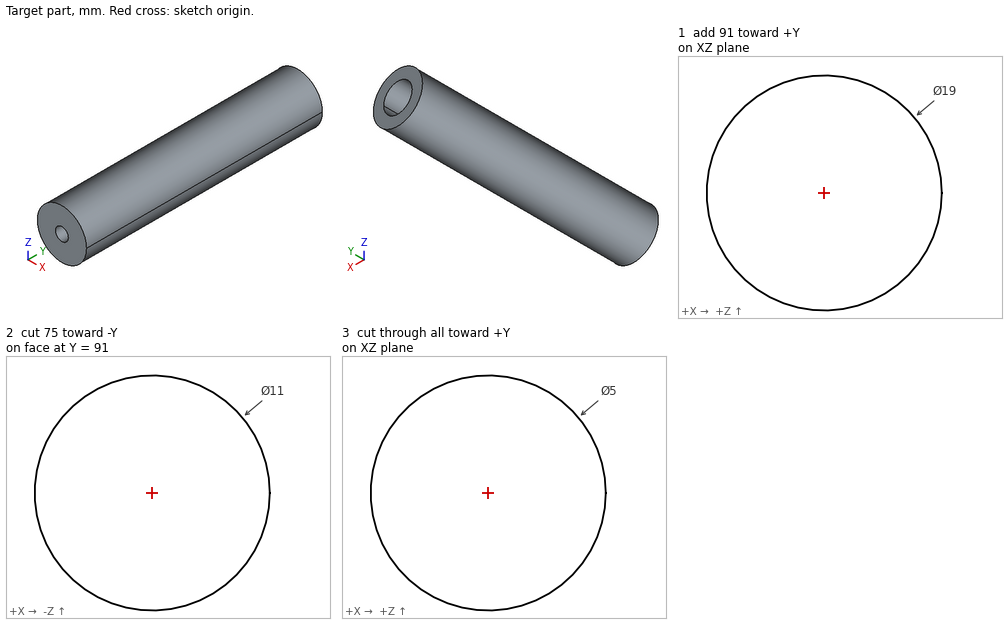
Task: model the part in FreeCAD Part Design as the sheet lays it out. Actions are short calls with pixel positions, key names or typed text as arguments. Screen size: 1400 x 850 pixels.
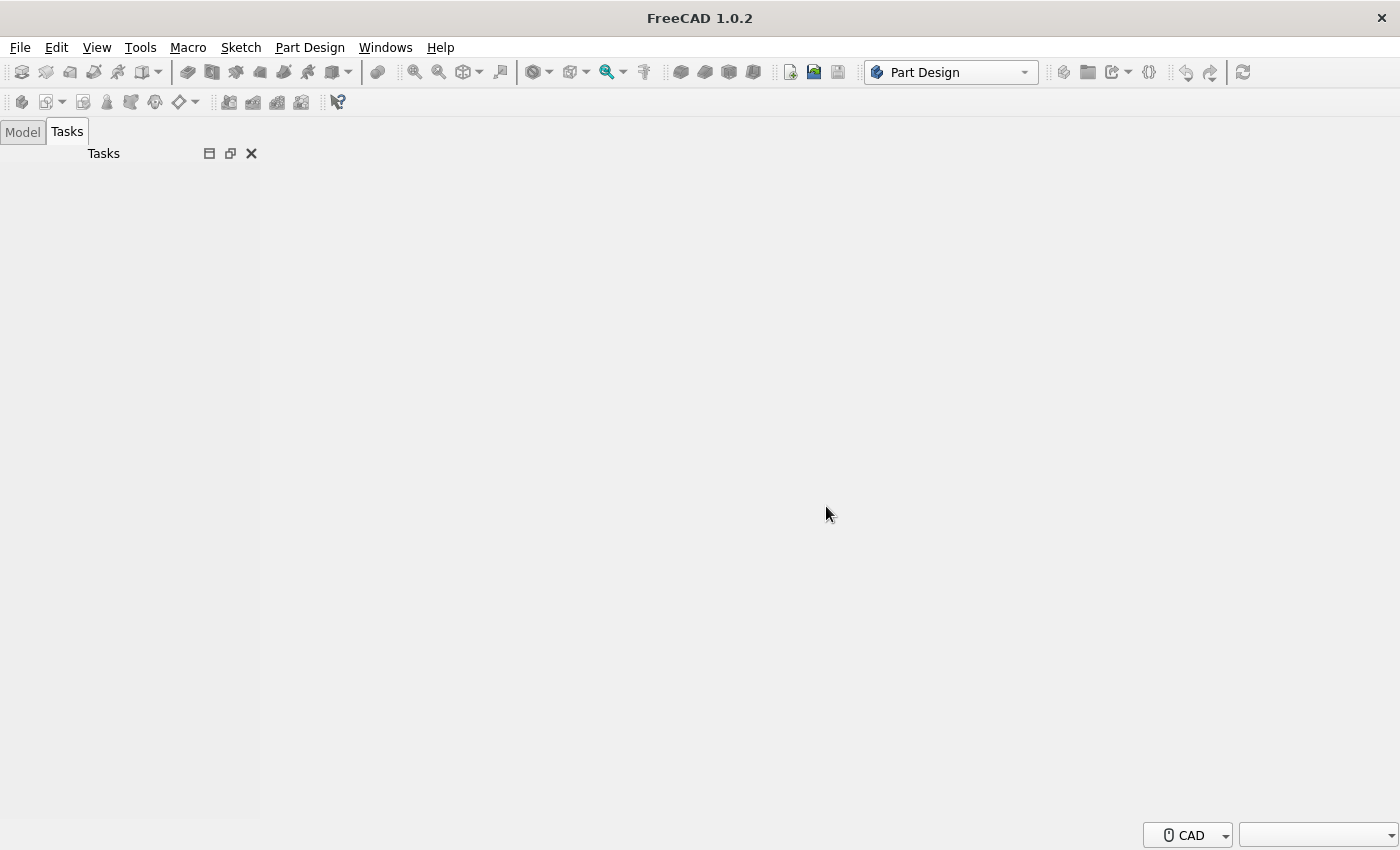
key(ctrl+n)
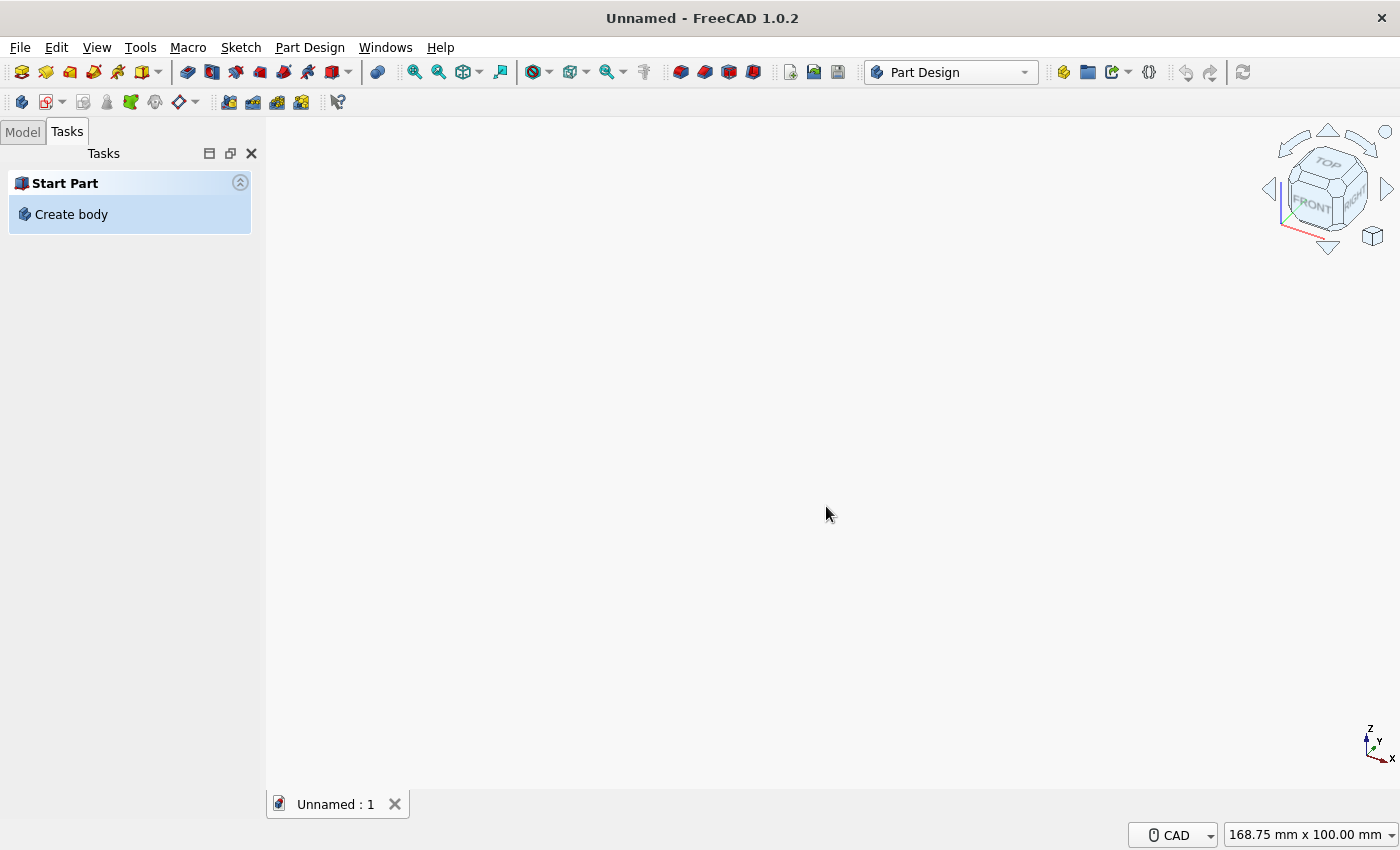
click(46, 102)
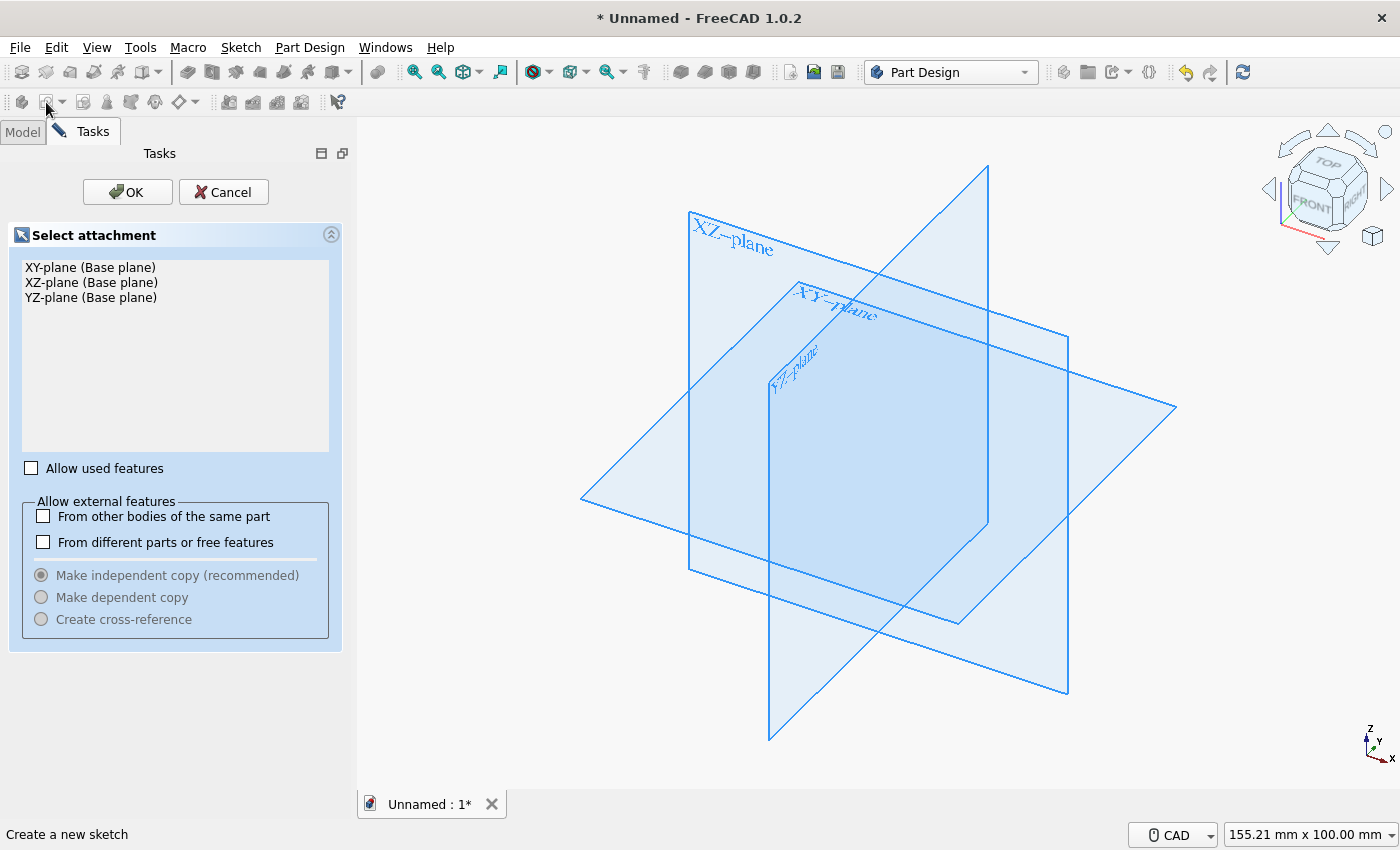
click(82, 282)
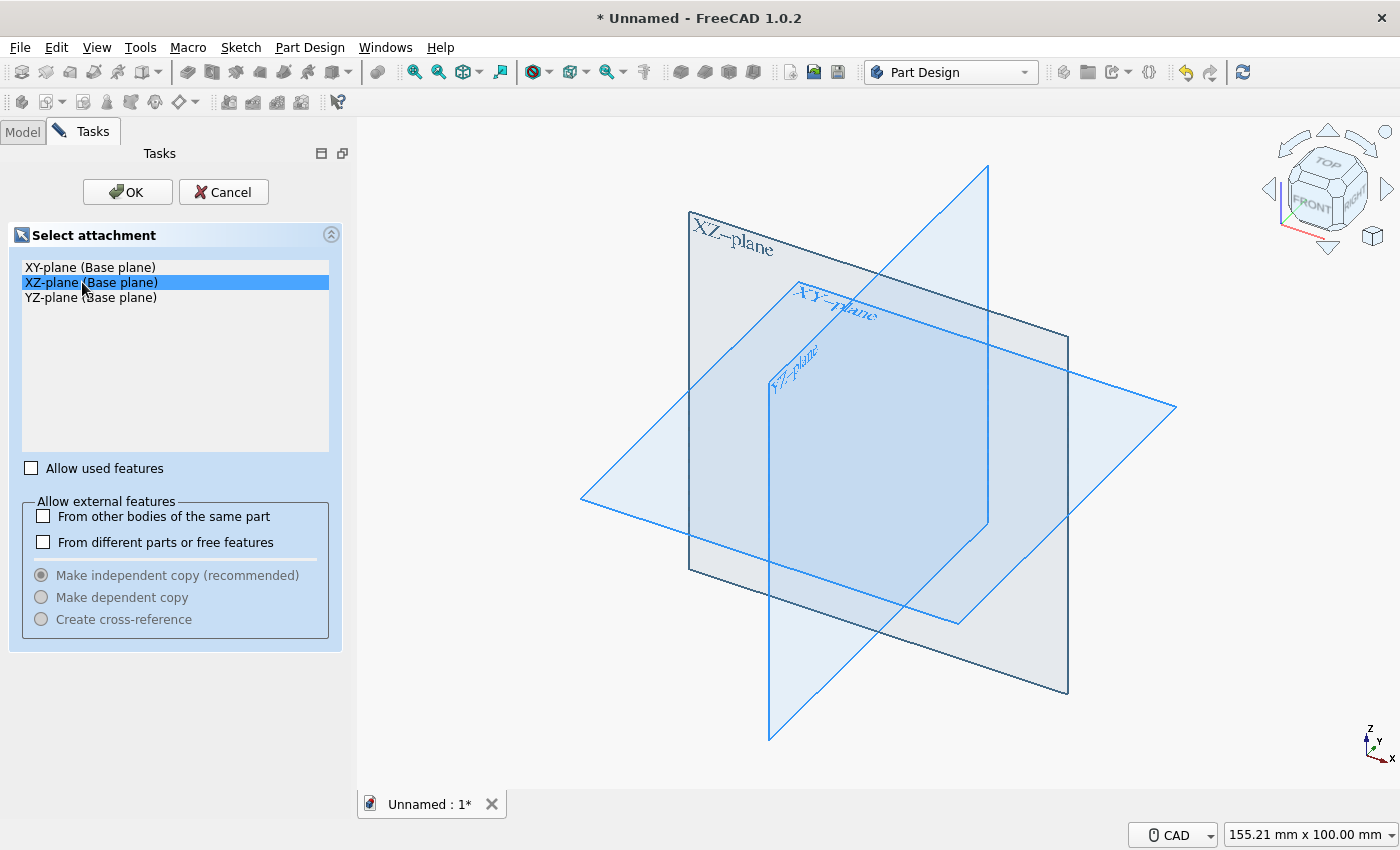
click(128, 192)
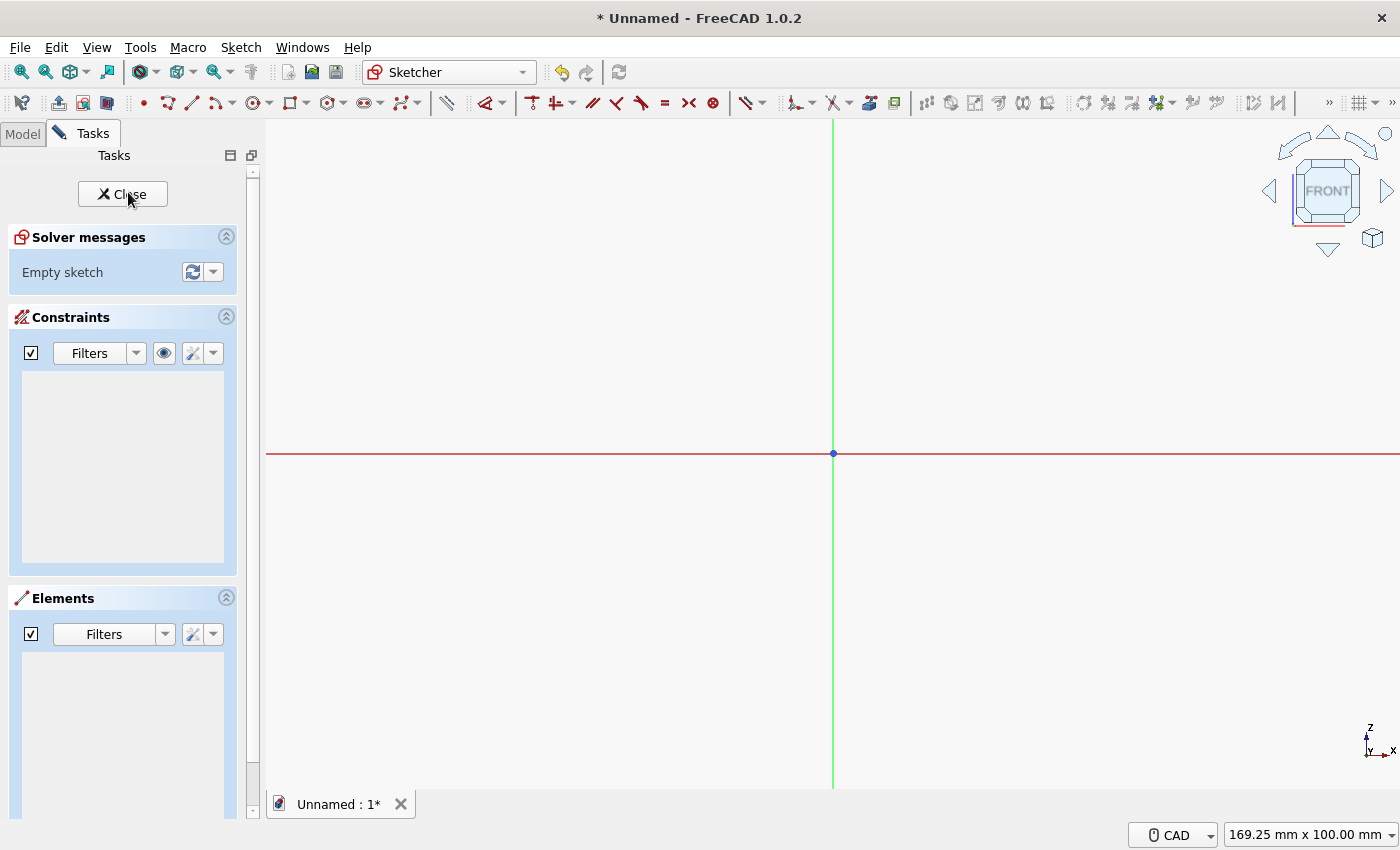
scroll(863, 454, up, 6)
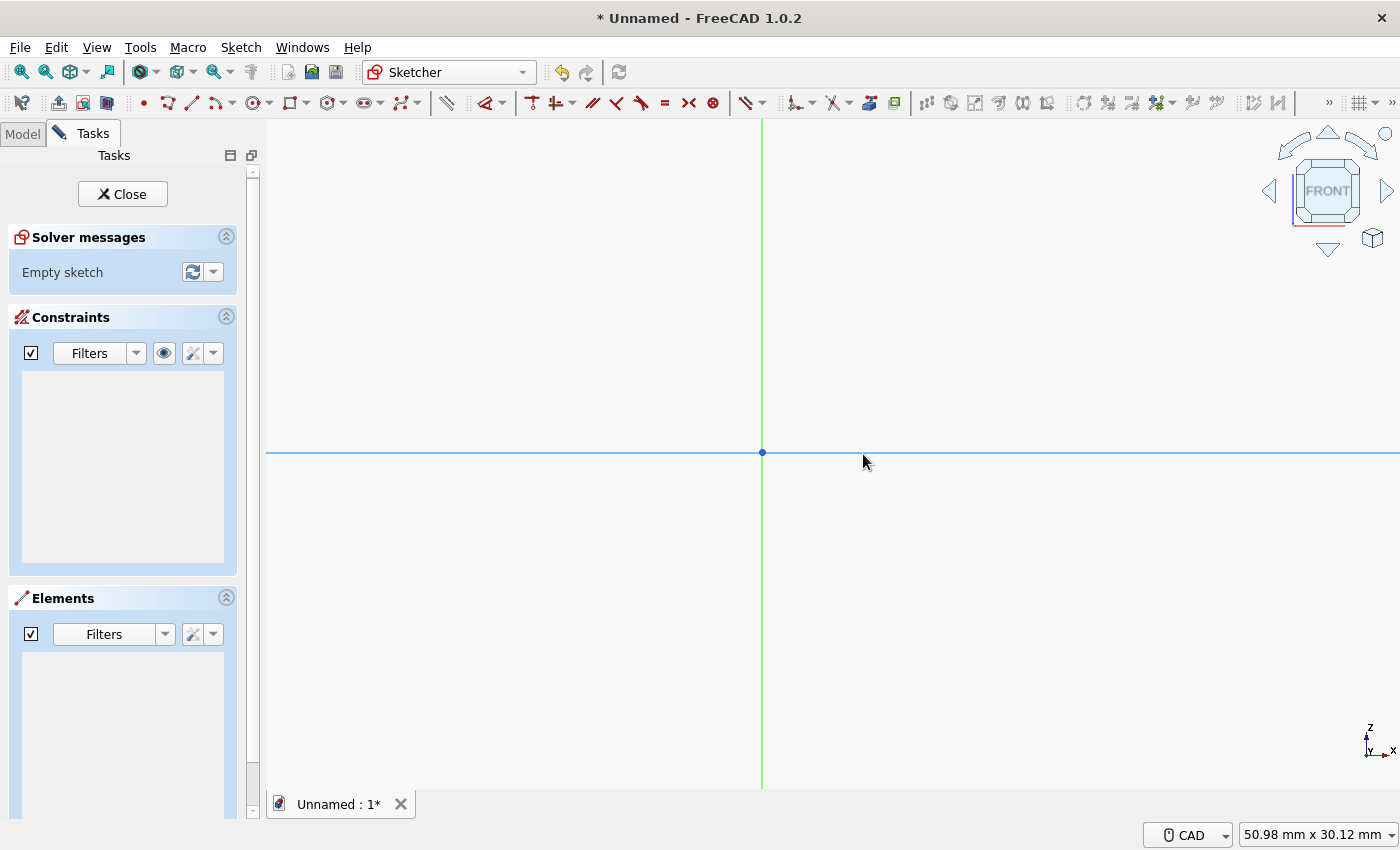
click(254, 104)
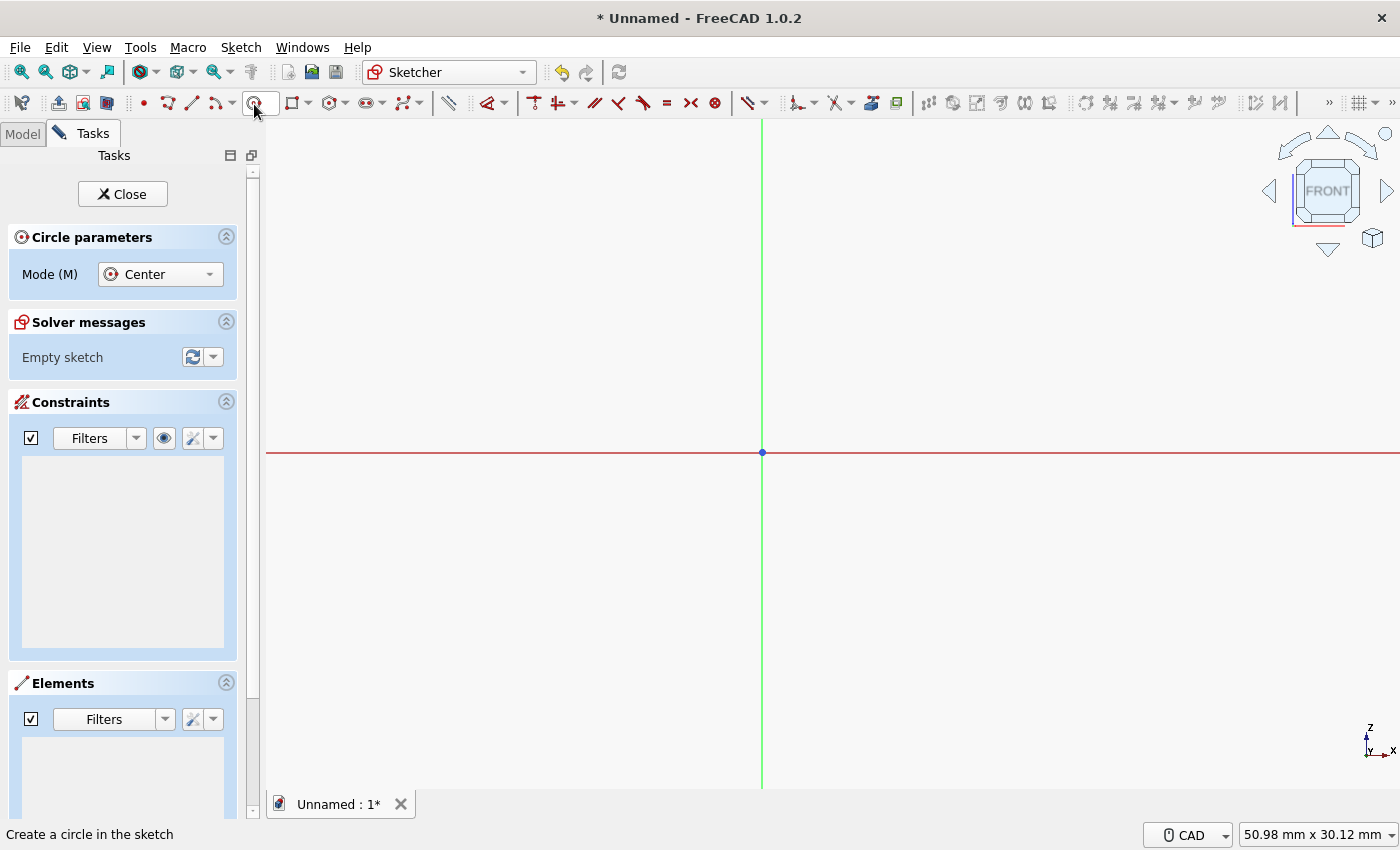
click(762, 453)
click(912, 303)
key(Escape)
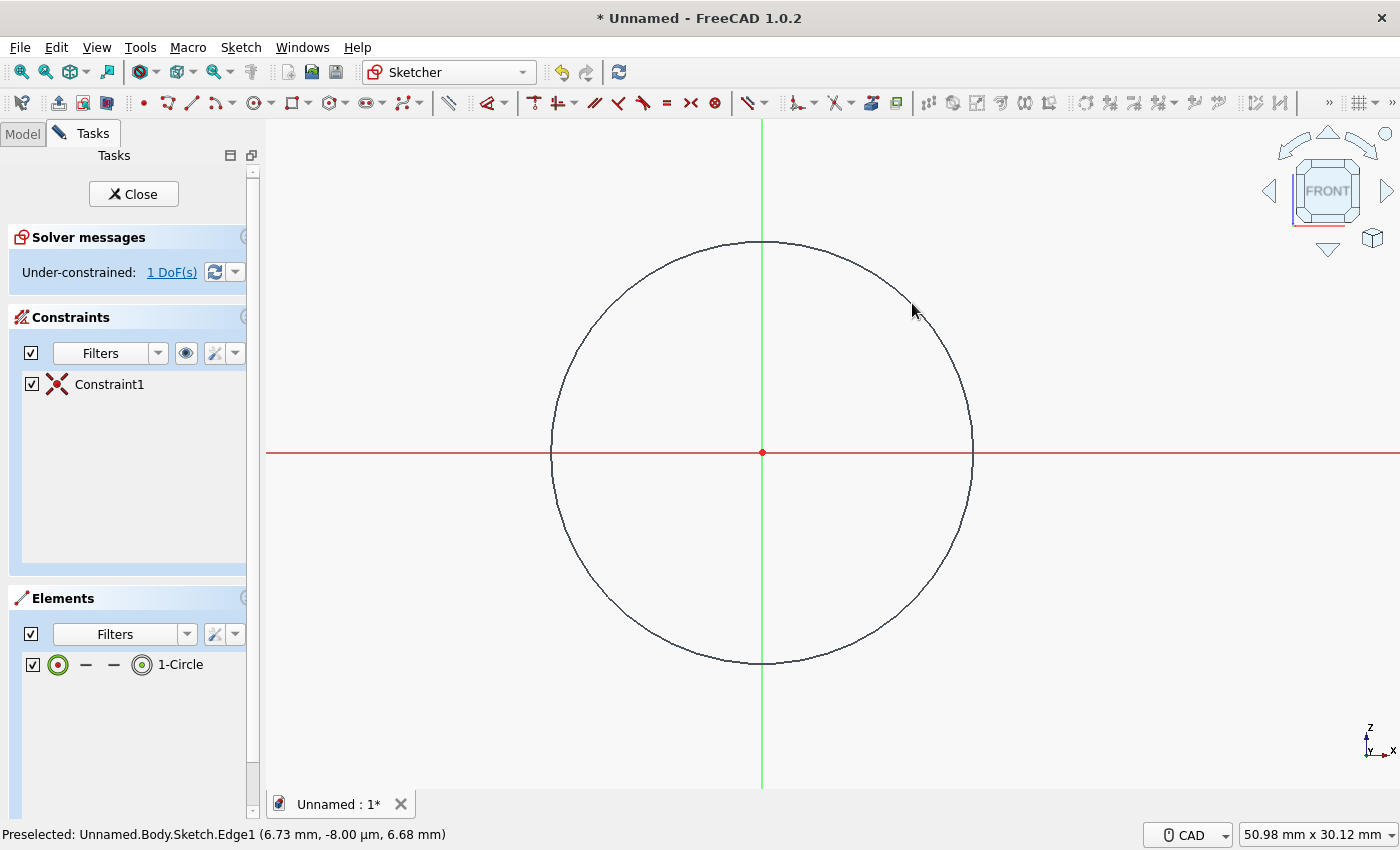
click(911, 303)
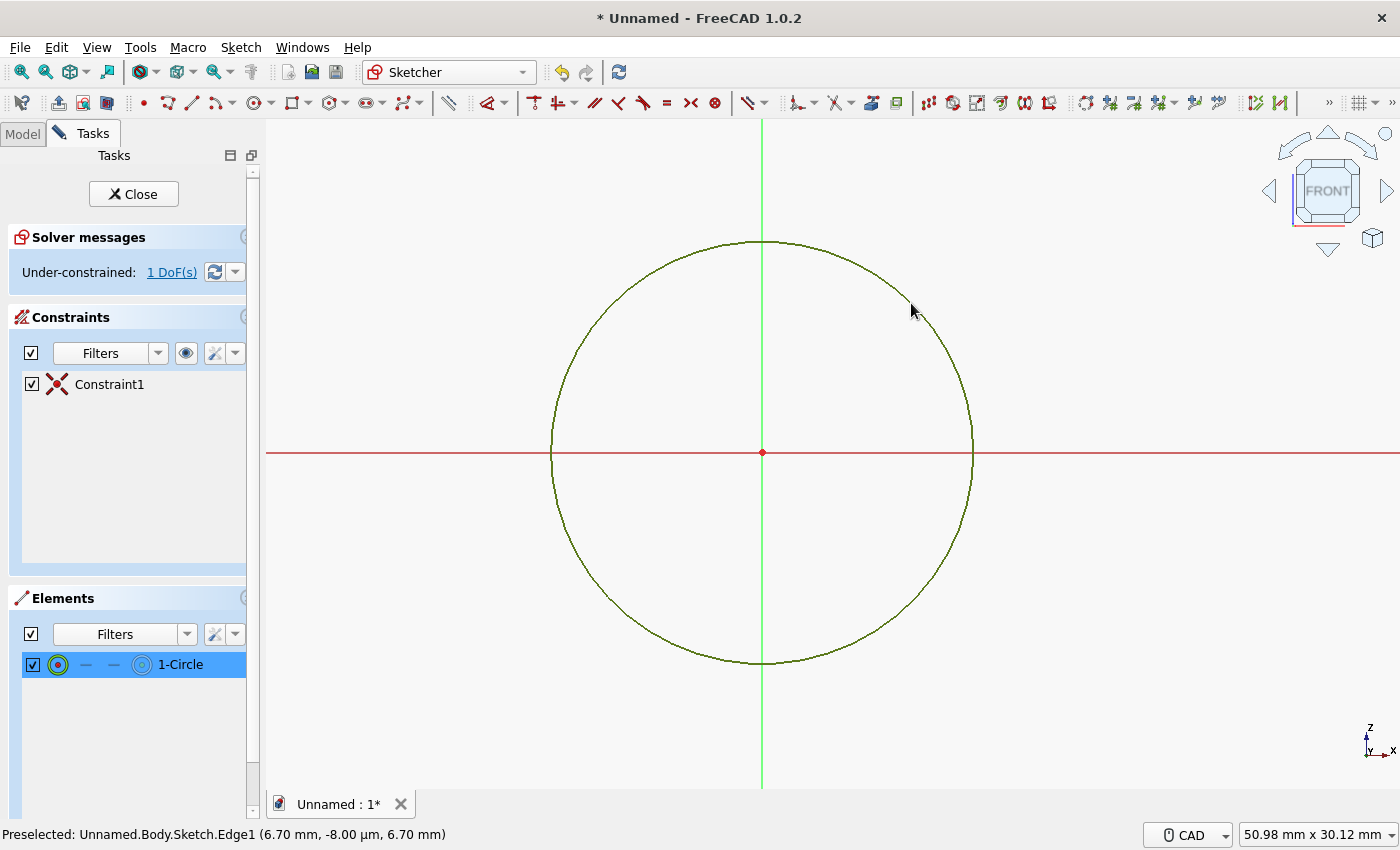
click(506, 104)